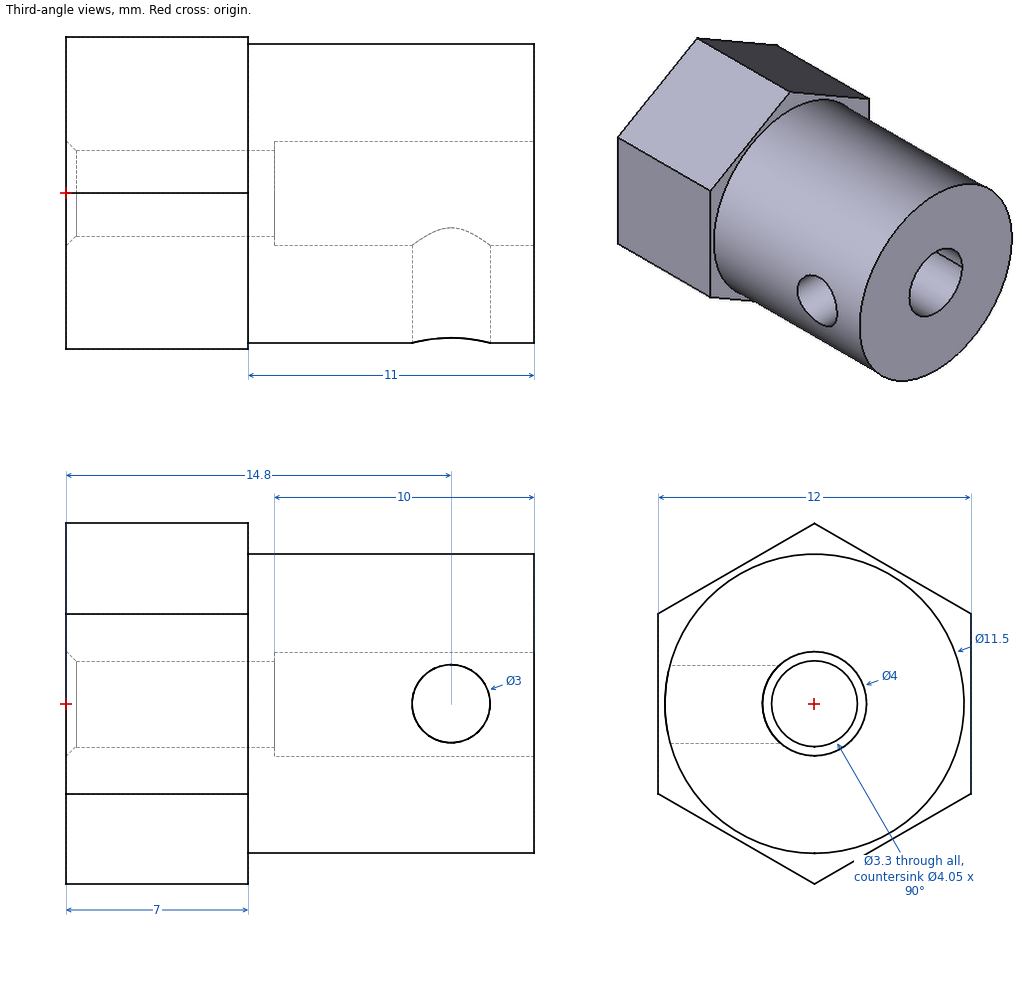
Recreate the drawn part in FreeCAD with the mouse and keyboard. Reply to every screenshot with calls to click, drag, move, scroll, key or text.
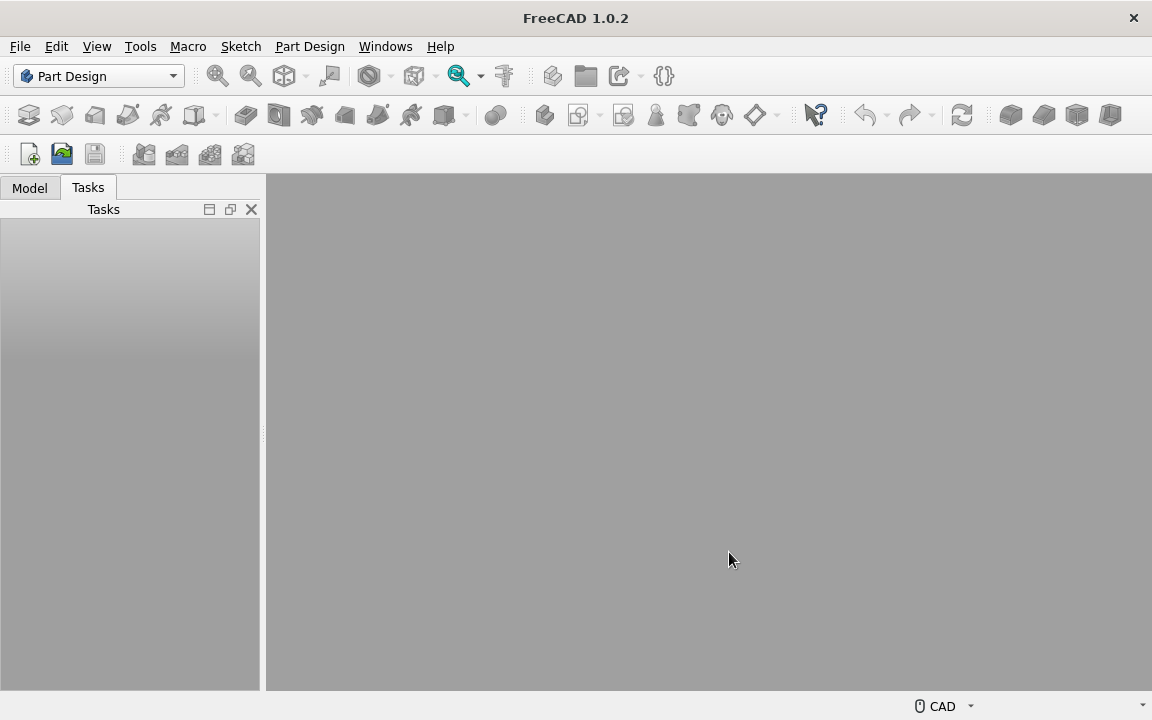
key(ctrl+n)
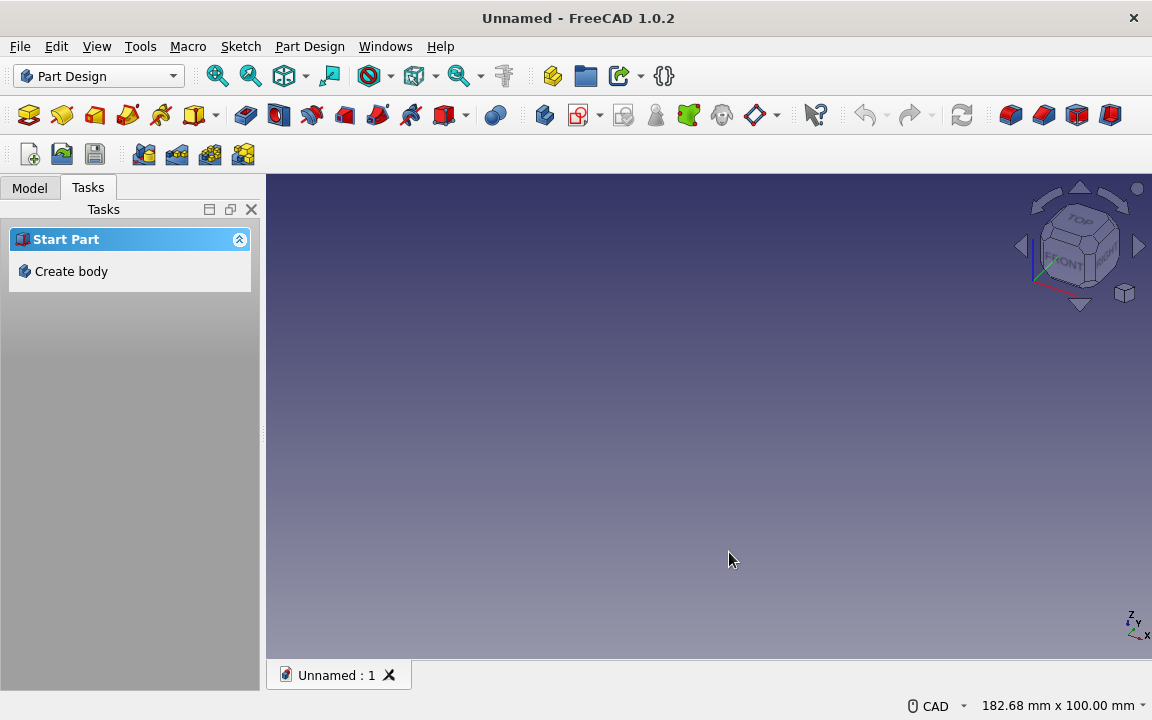
click(578, 116)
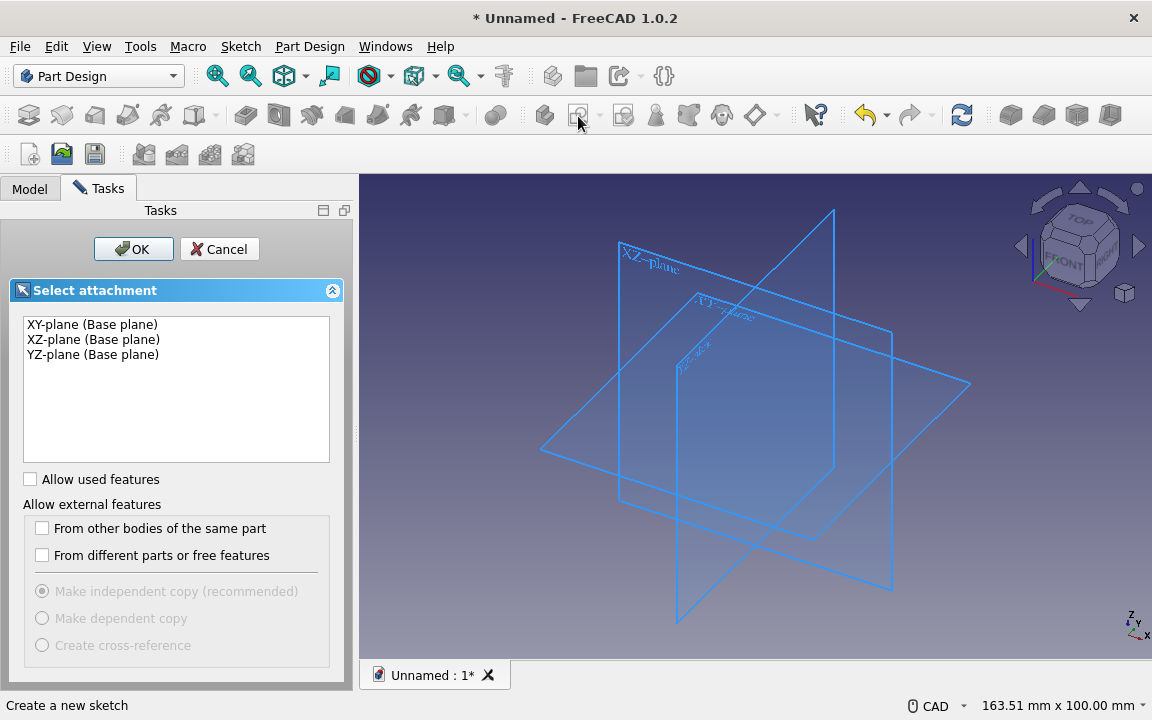
click(84, 354)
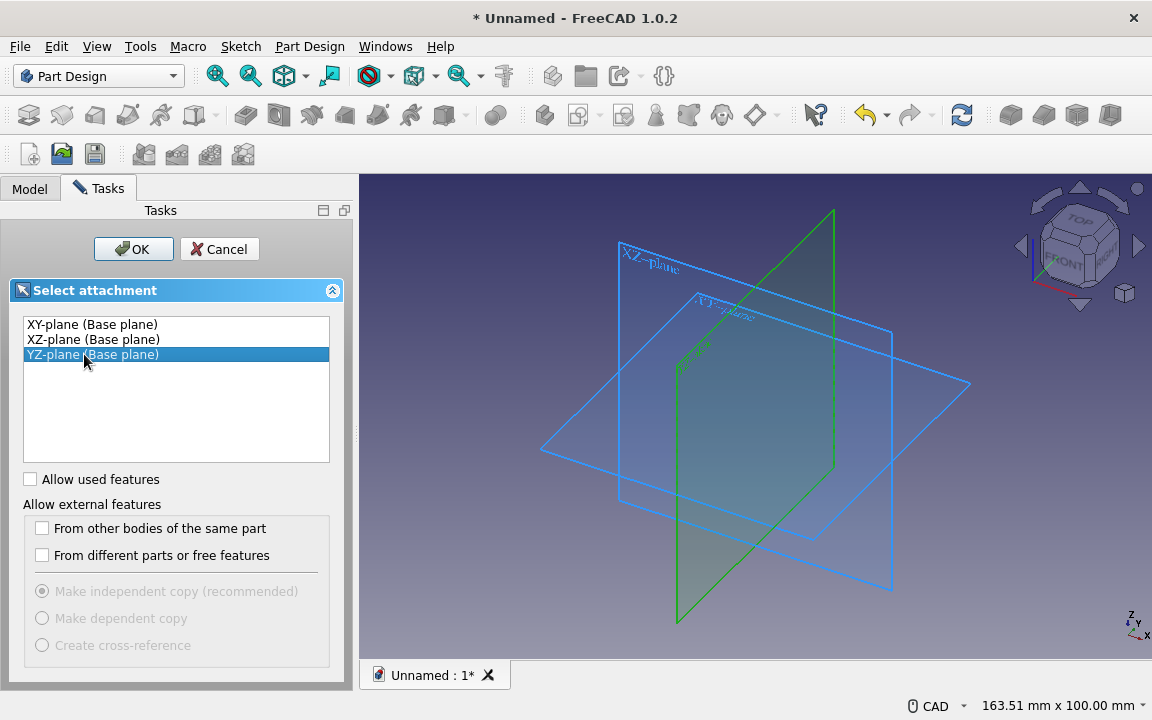
click(134, 249)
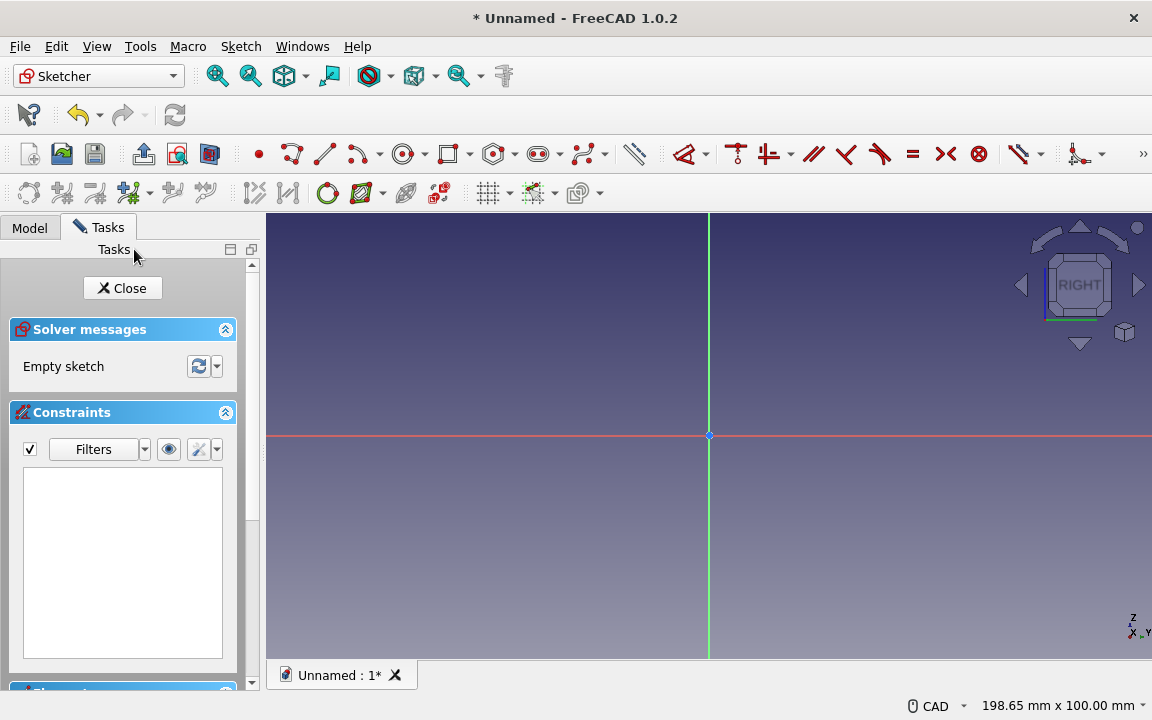
scroll(731, 436, up, 7)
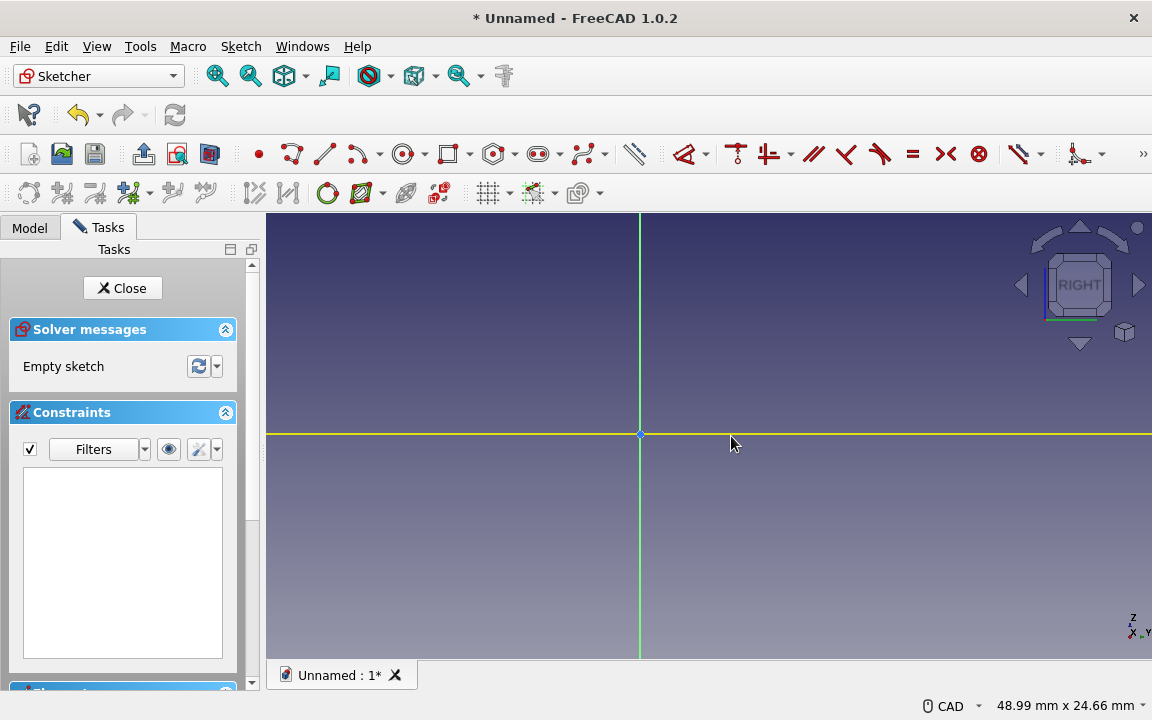
key(g)
key(p)
key(6)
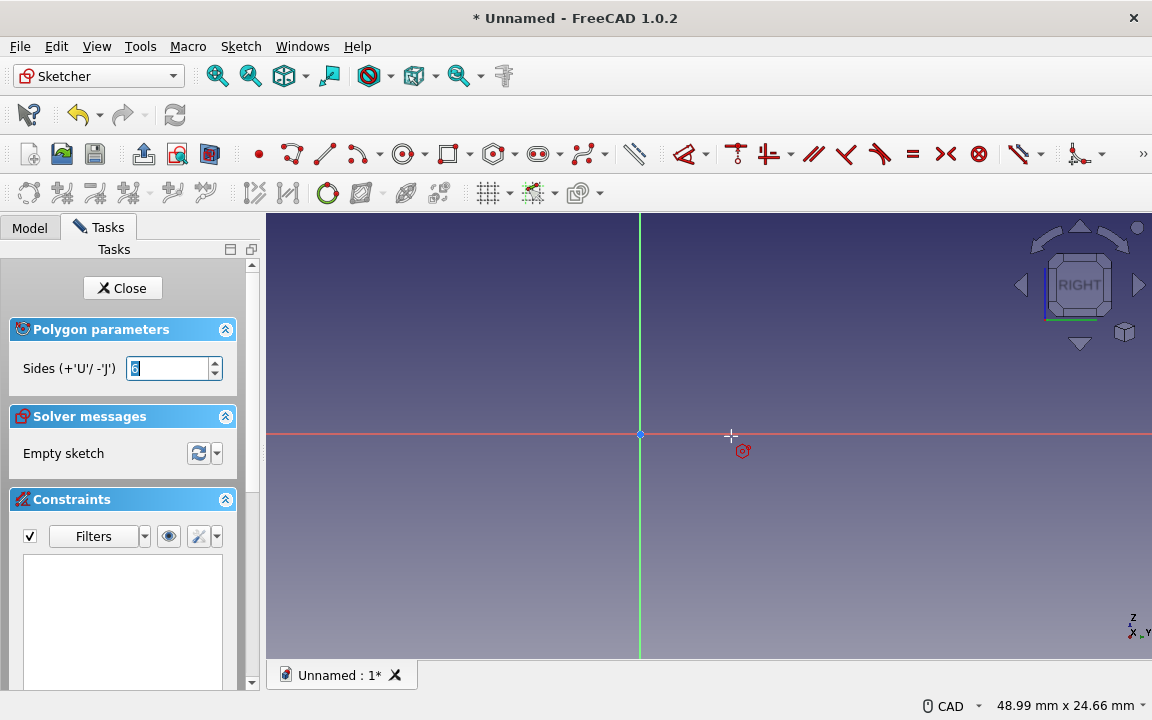
click(640, 434)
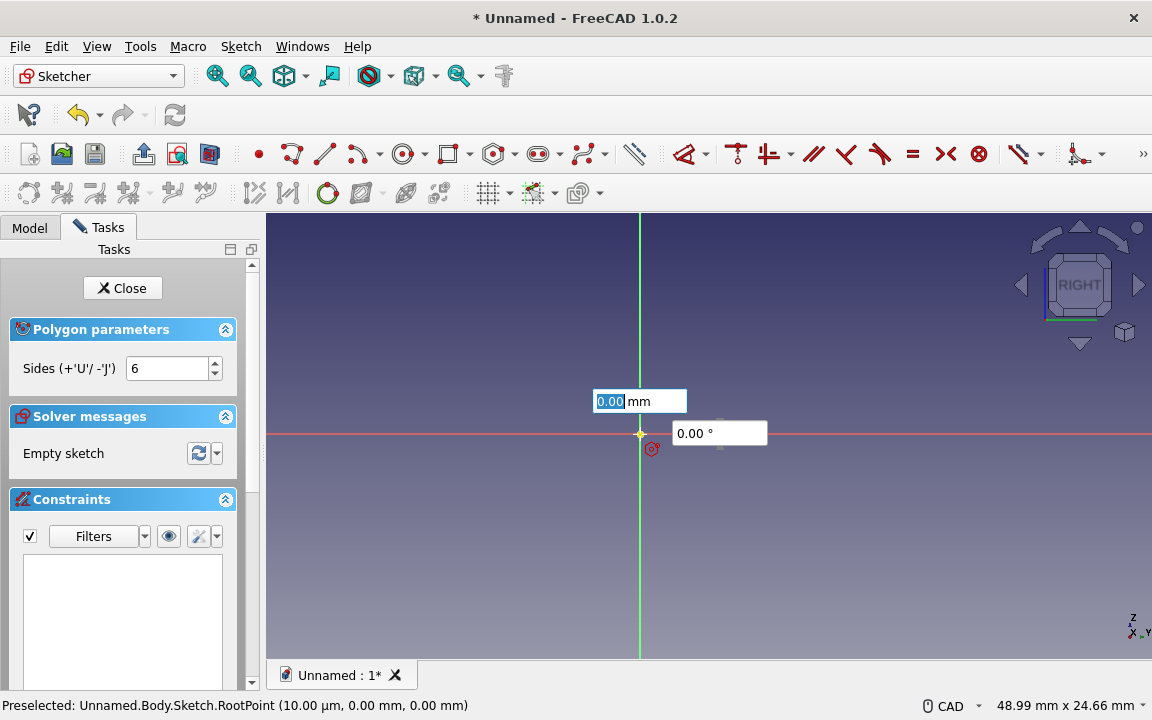
click(640, 560)
right_click(640, 560)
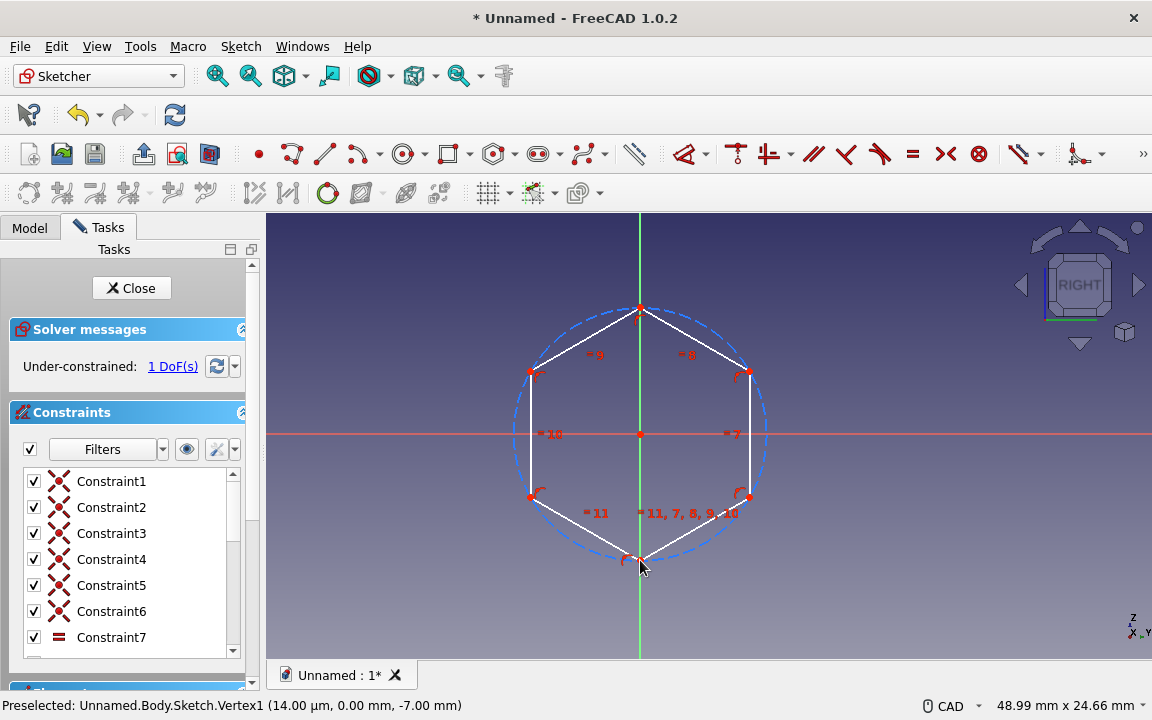
key(d)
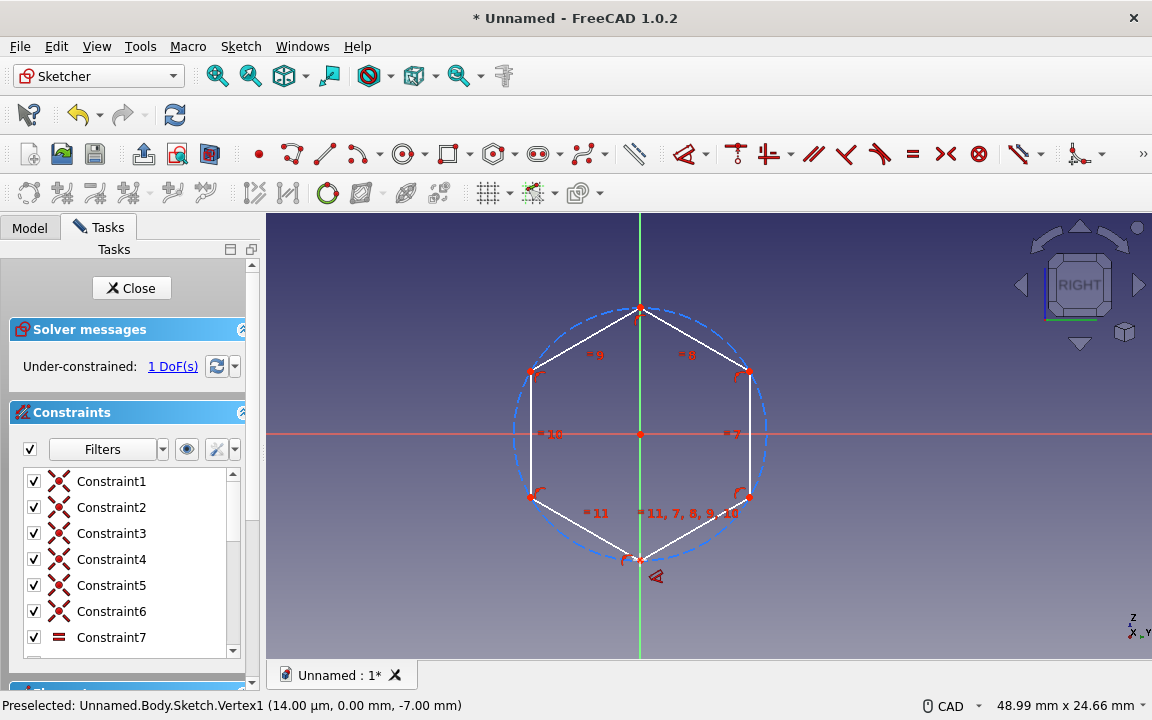
click(531, 371)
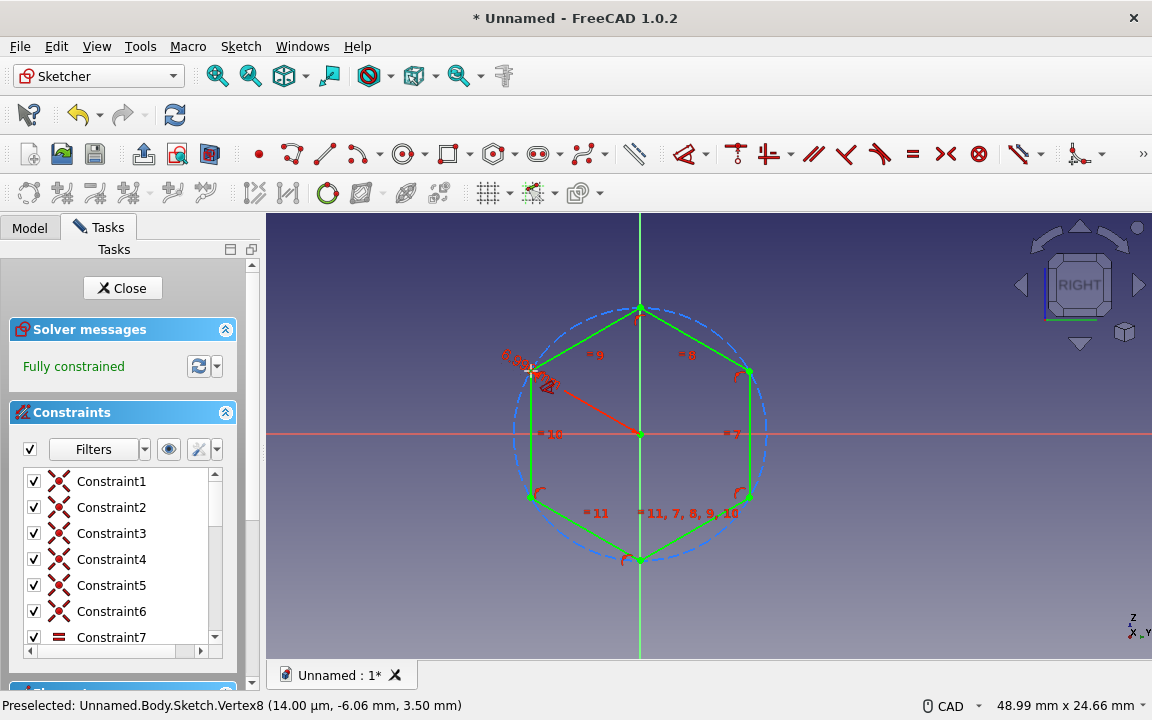
click(750, 498)
click(563, 556)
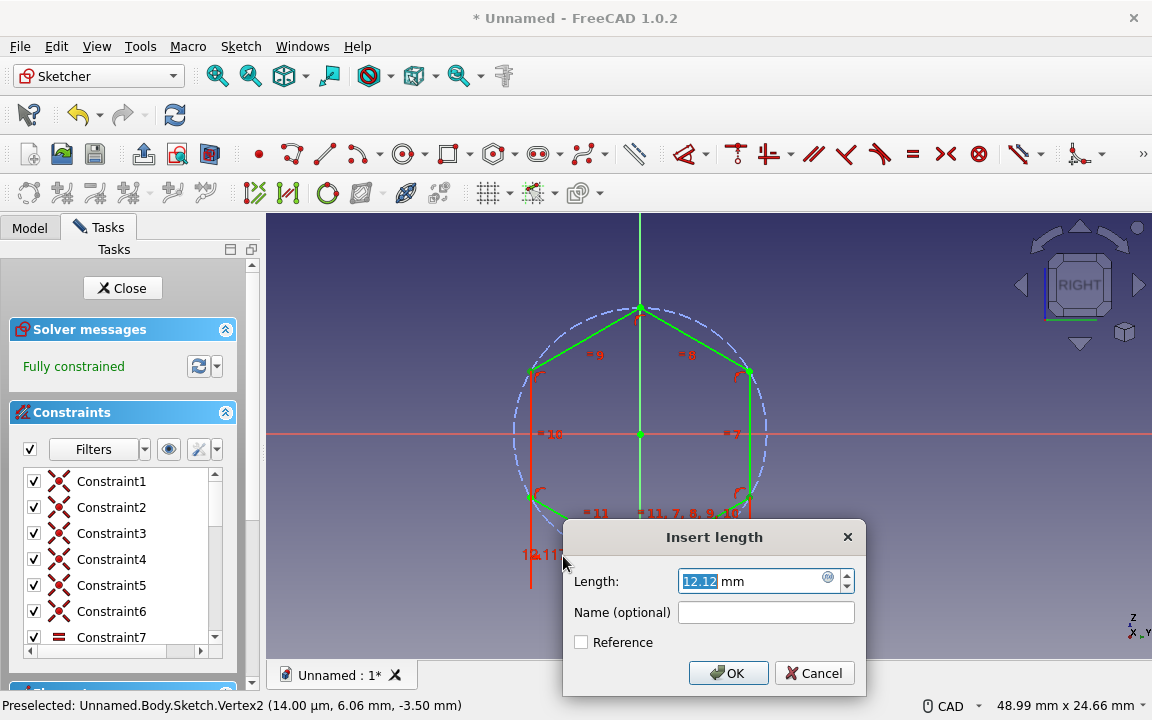
text(12)
key(Return)
key(Escape)